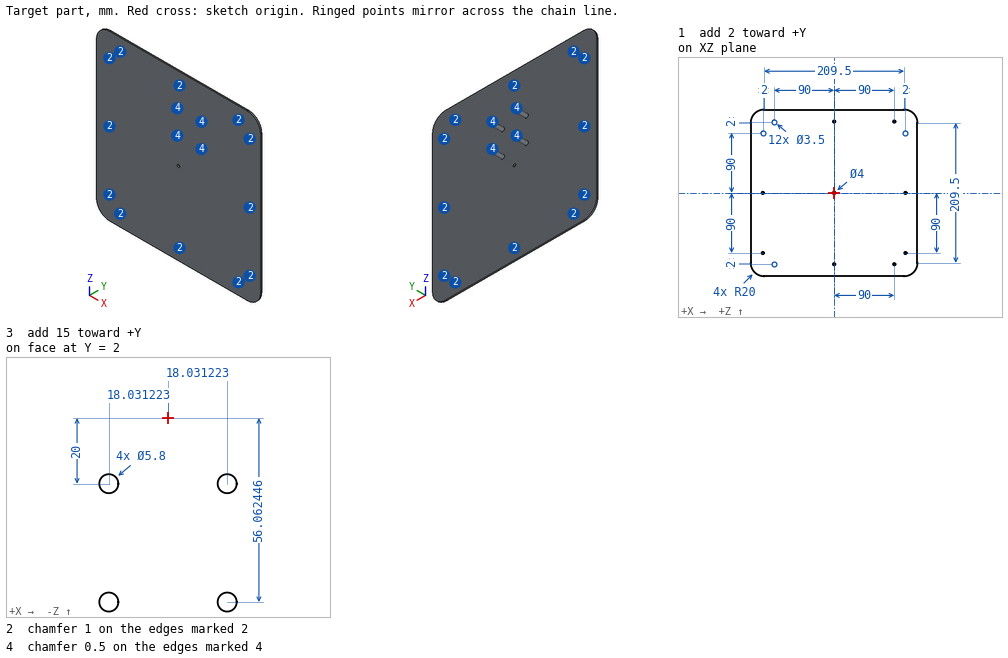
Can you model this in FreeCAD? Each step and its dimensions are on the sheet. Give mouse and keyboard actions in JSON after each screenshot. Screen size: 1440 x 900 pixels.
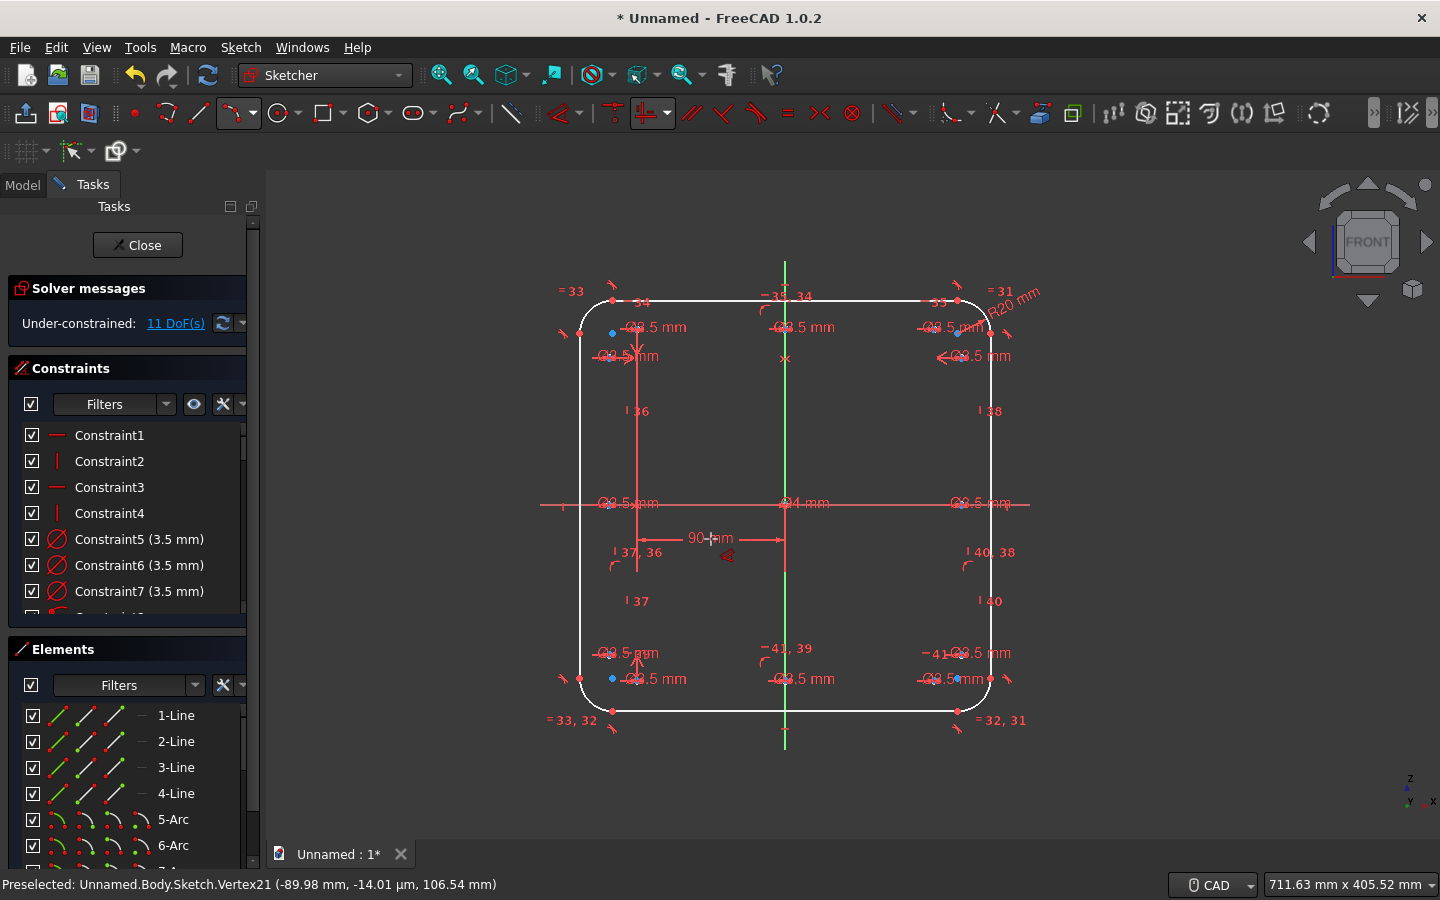
{"action": "left_click", "coordinate": [609, 358]}
{"action": "left_click", "coordinate": [819, 432]}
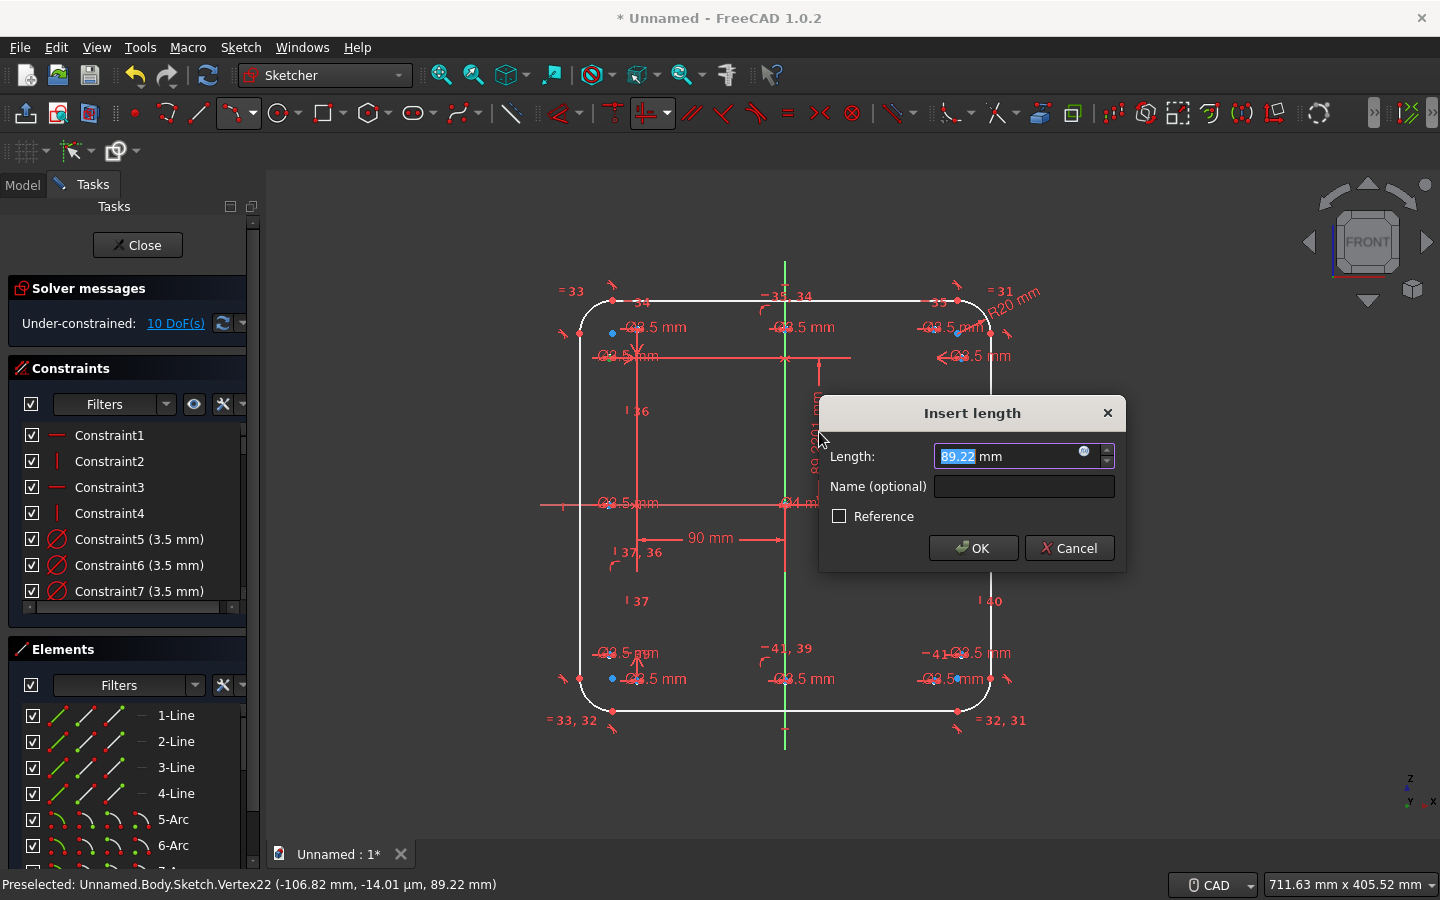
{"action": "type", "text": "90"}
{"action": "key", "text": "Return"}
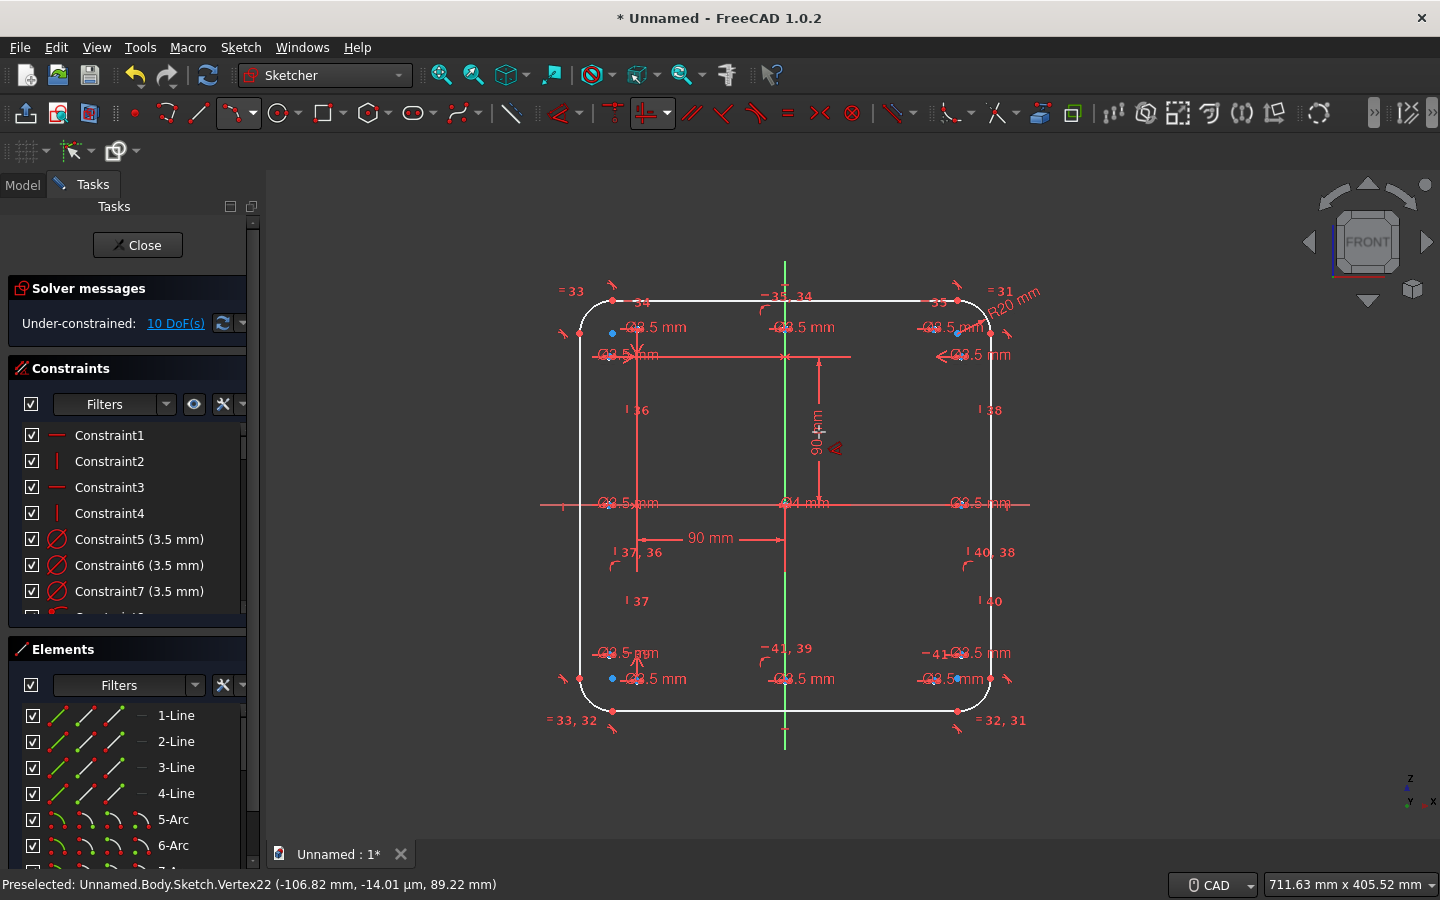
{"action": "left_click", "coordinate": [934, 329]}
{"action": "left_click", "coordinate": [860, 539]}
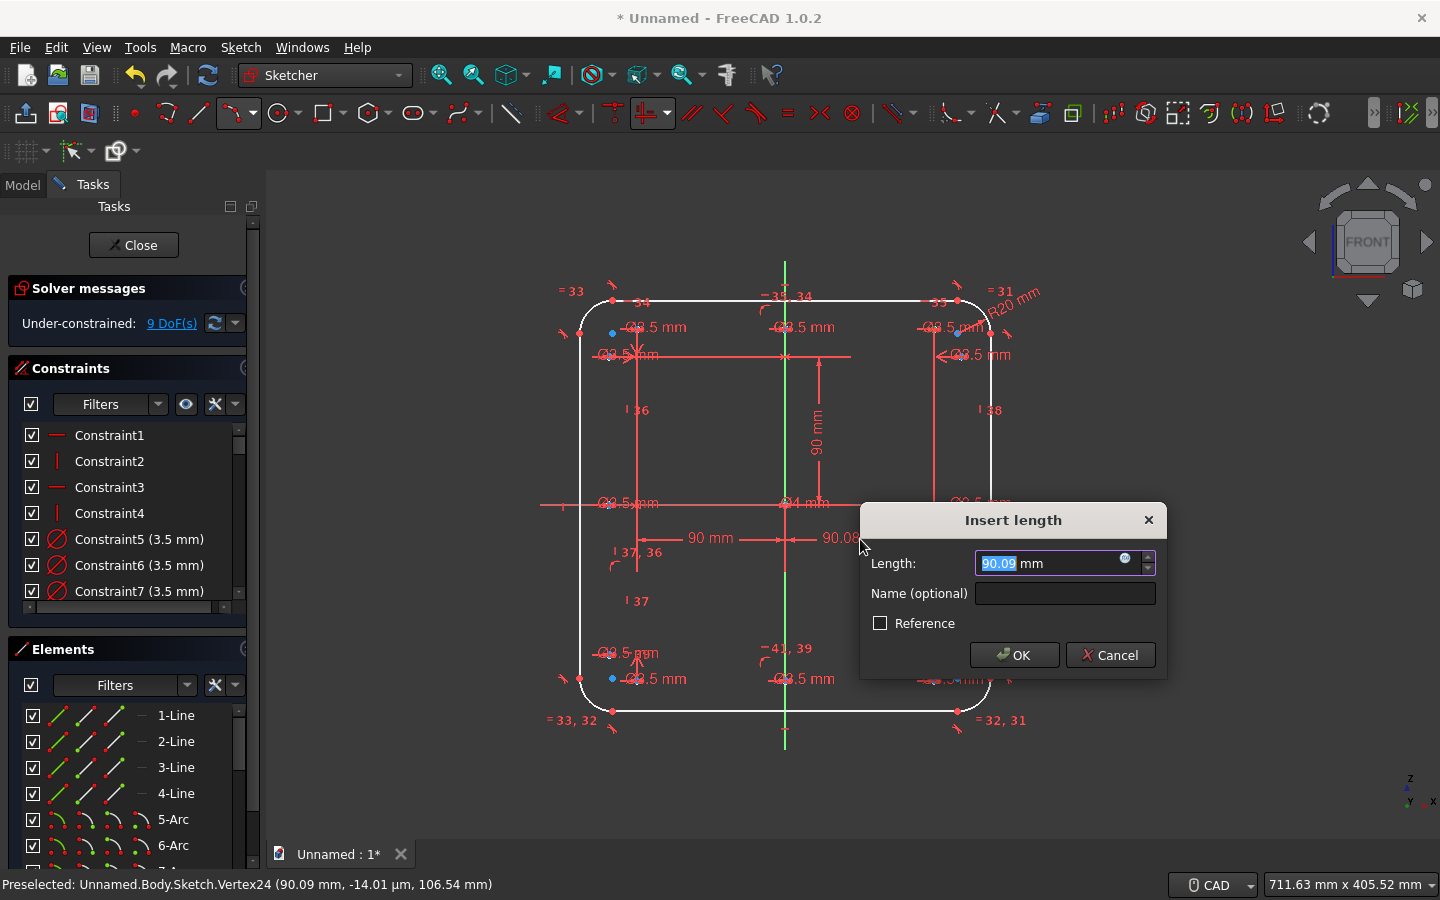
{"action": "type", "text": "90"}
{"action": "key", "text": "Return"}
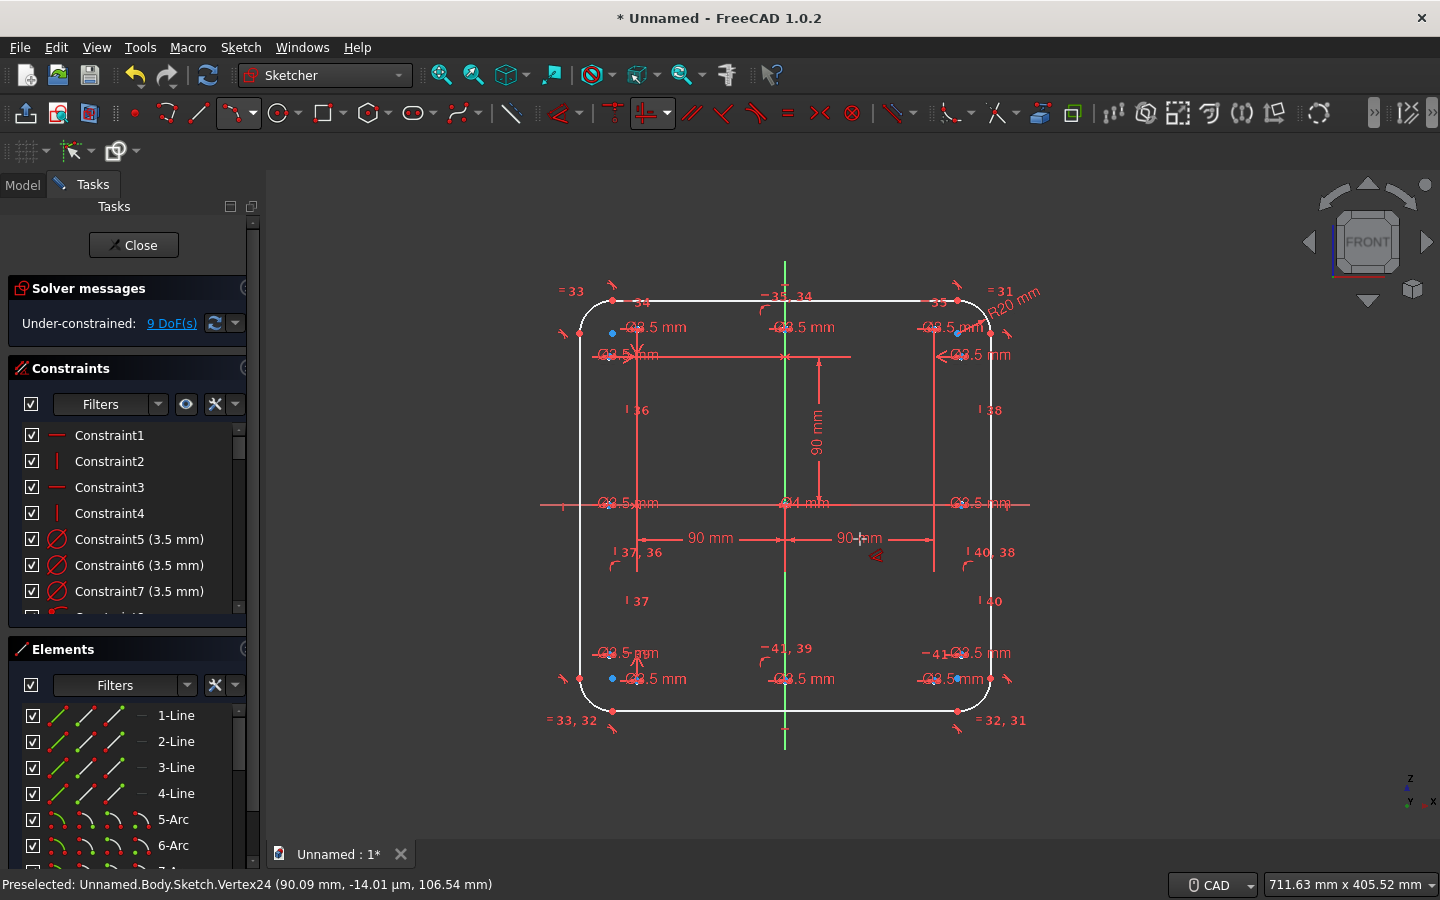
{"action": "left_click", "coordinate": [609, 655]}
{"action": "left_click", "coordinate": [819, 580]}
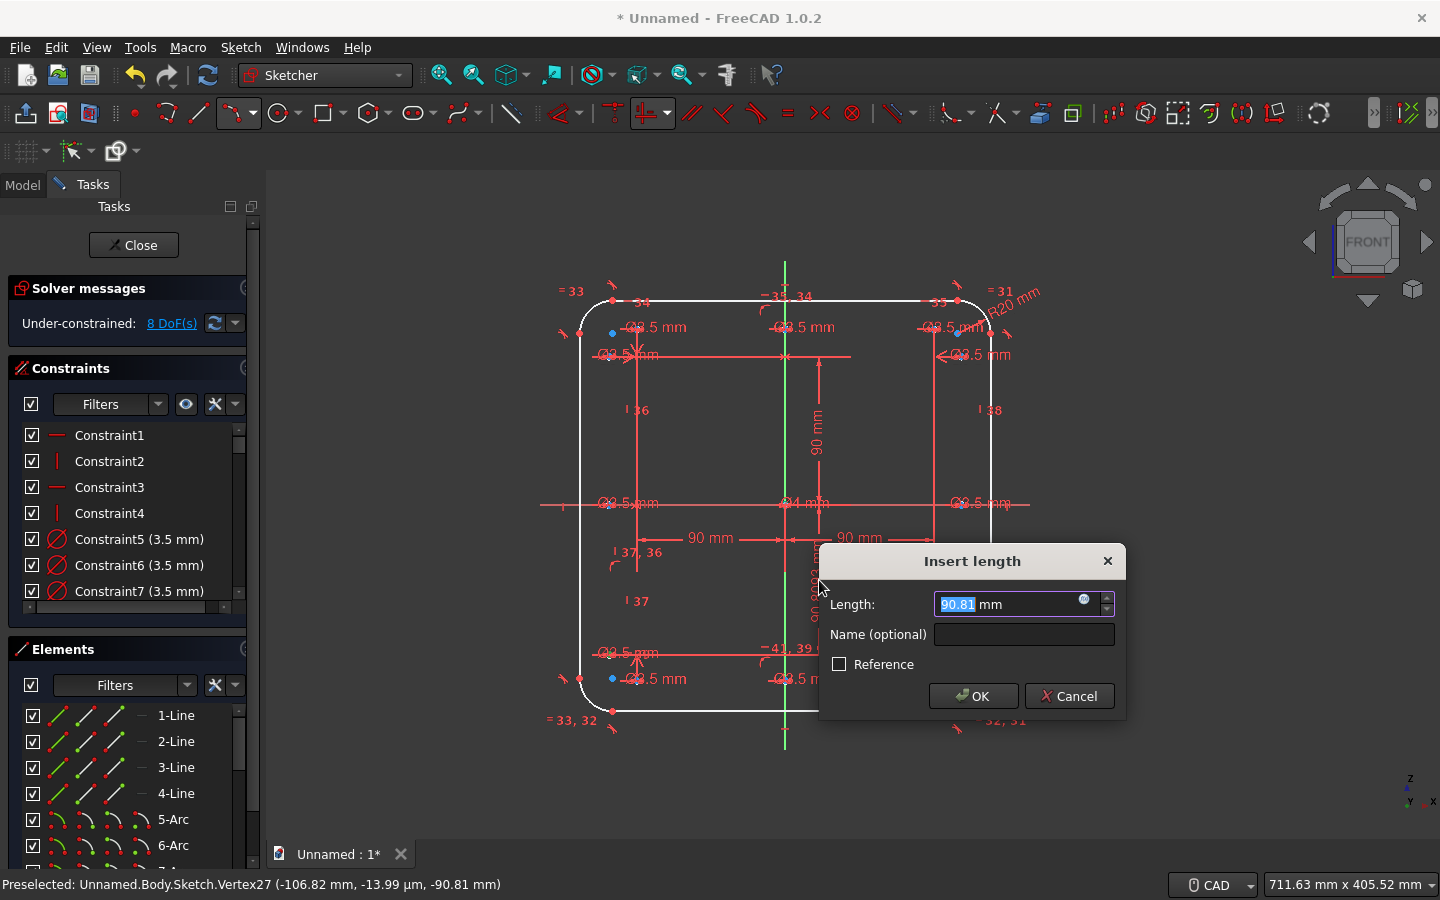
{"action": "type", "text": "90"}
{"action": "key", "text": "Return"}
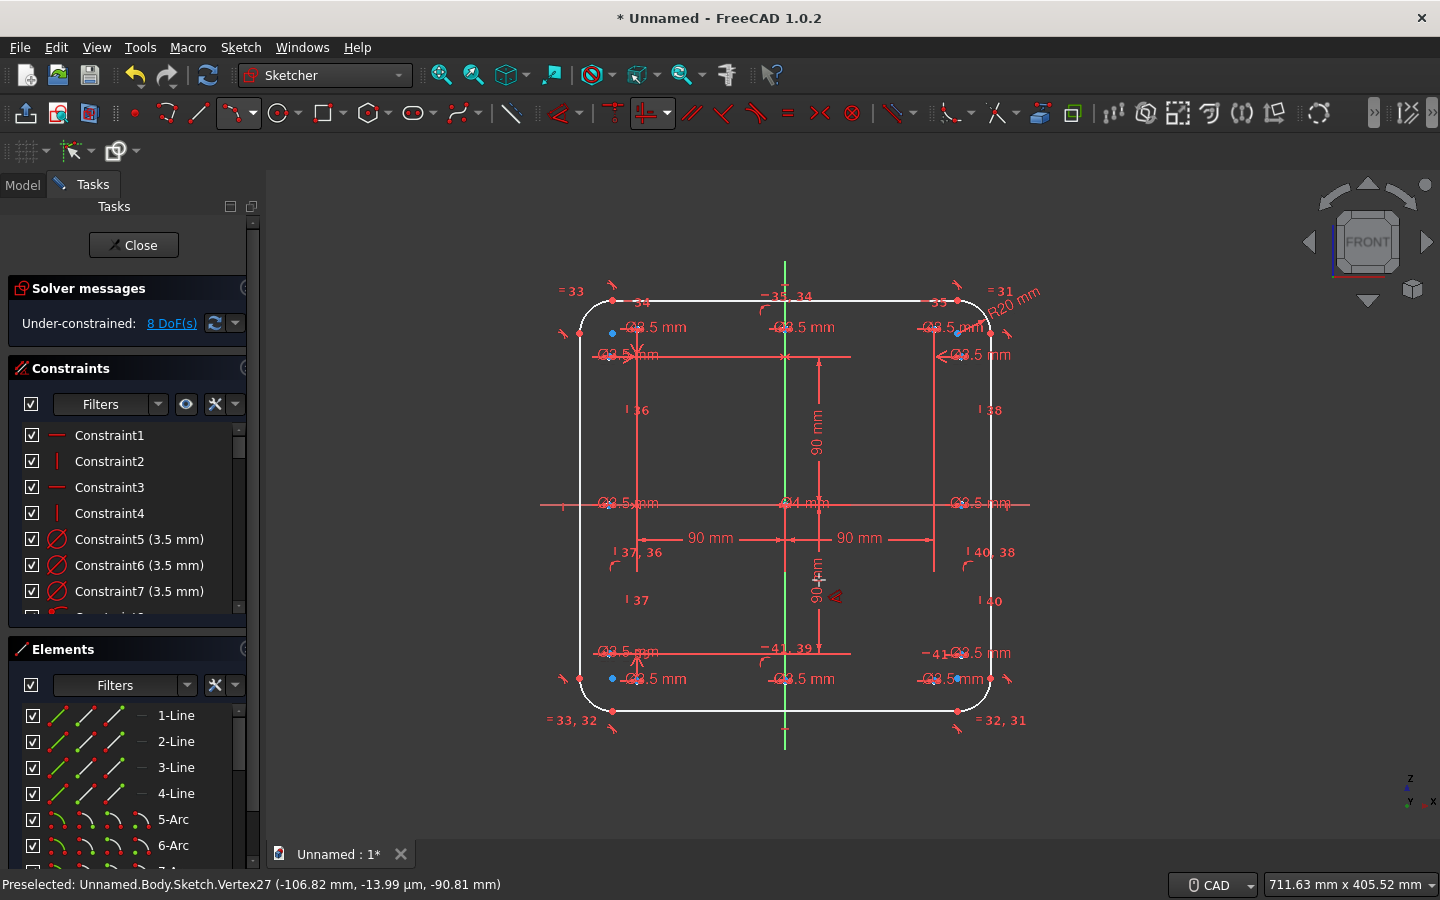
{"action": "left_click", "coordinate": [962, 655]}
{"action": "left_click", "coordinate": [751, 615]}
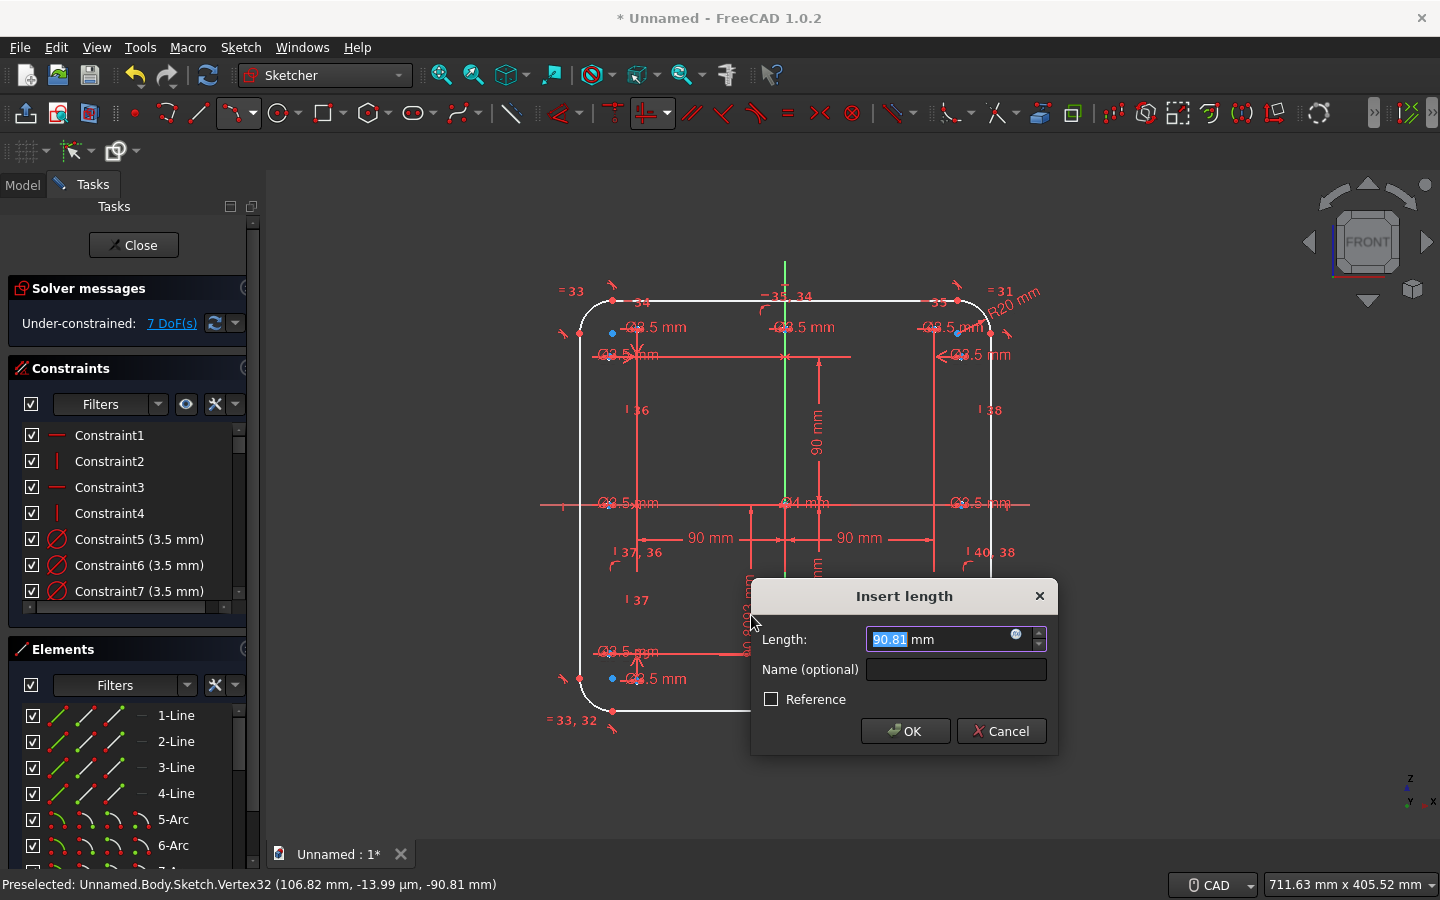
{"action": "type", "text": "90"}
{"action": "key", "text": "Return"}